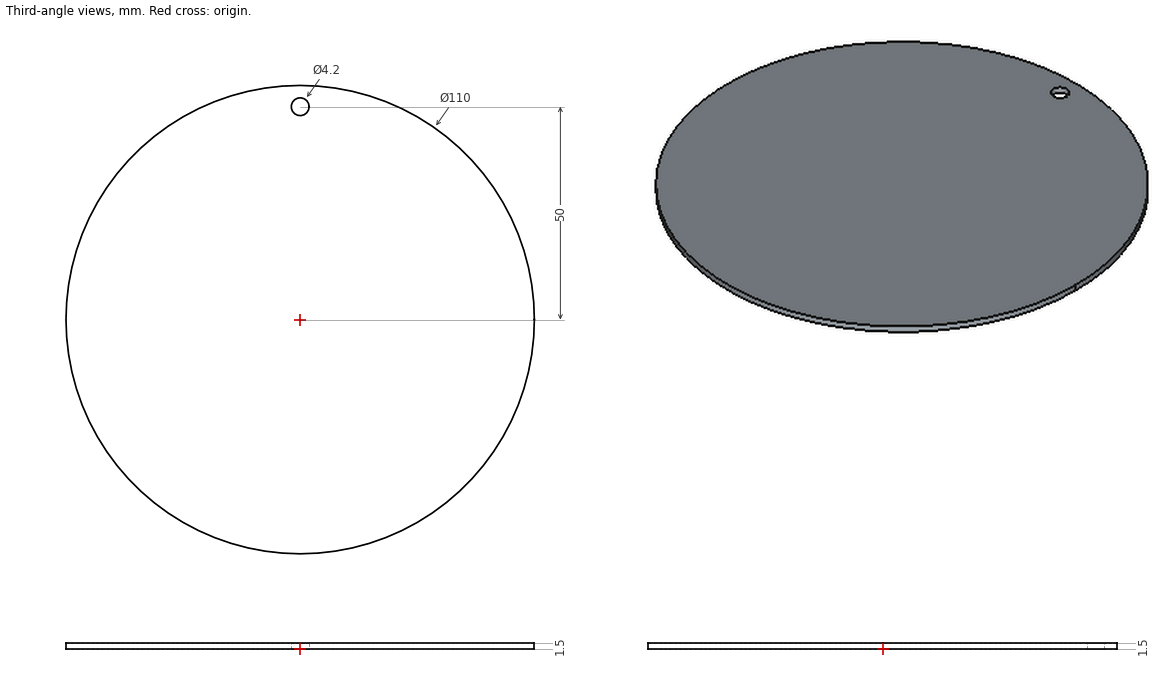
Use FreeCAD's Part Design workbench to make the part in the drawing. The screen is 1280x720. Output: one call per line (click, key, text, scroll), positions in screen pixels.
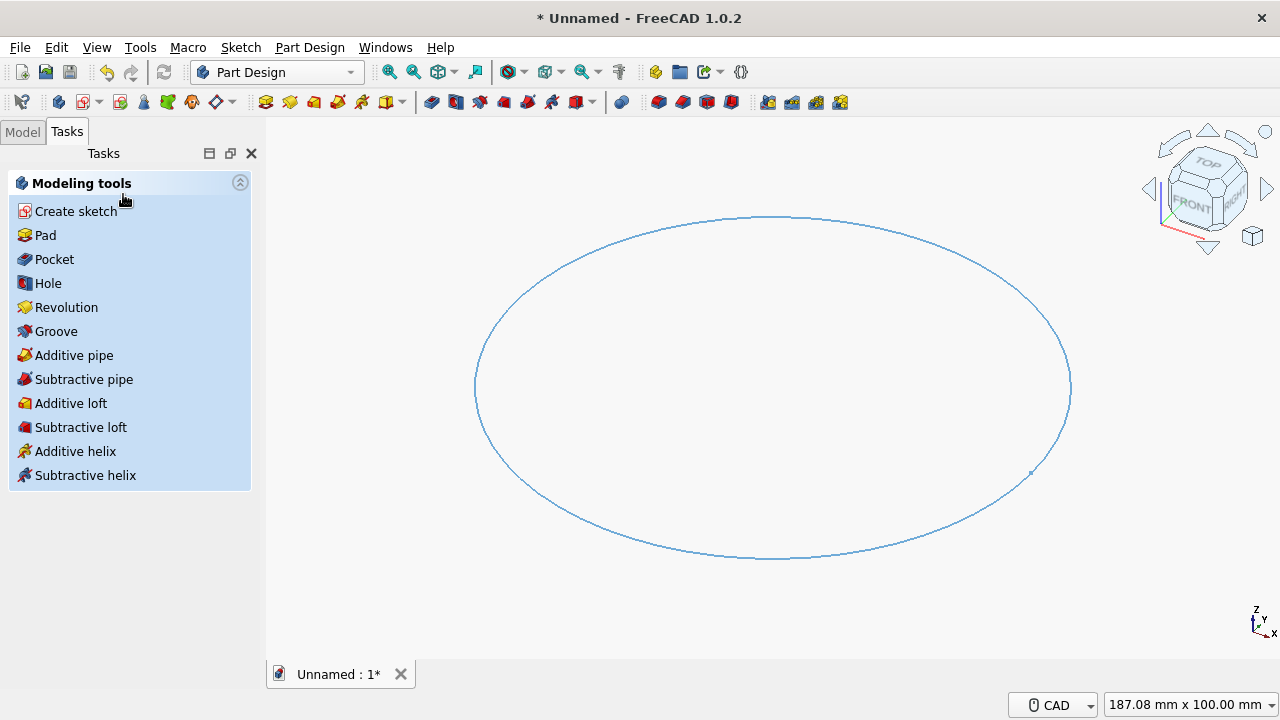
click(266, 102)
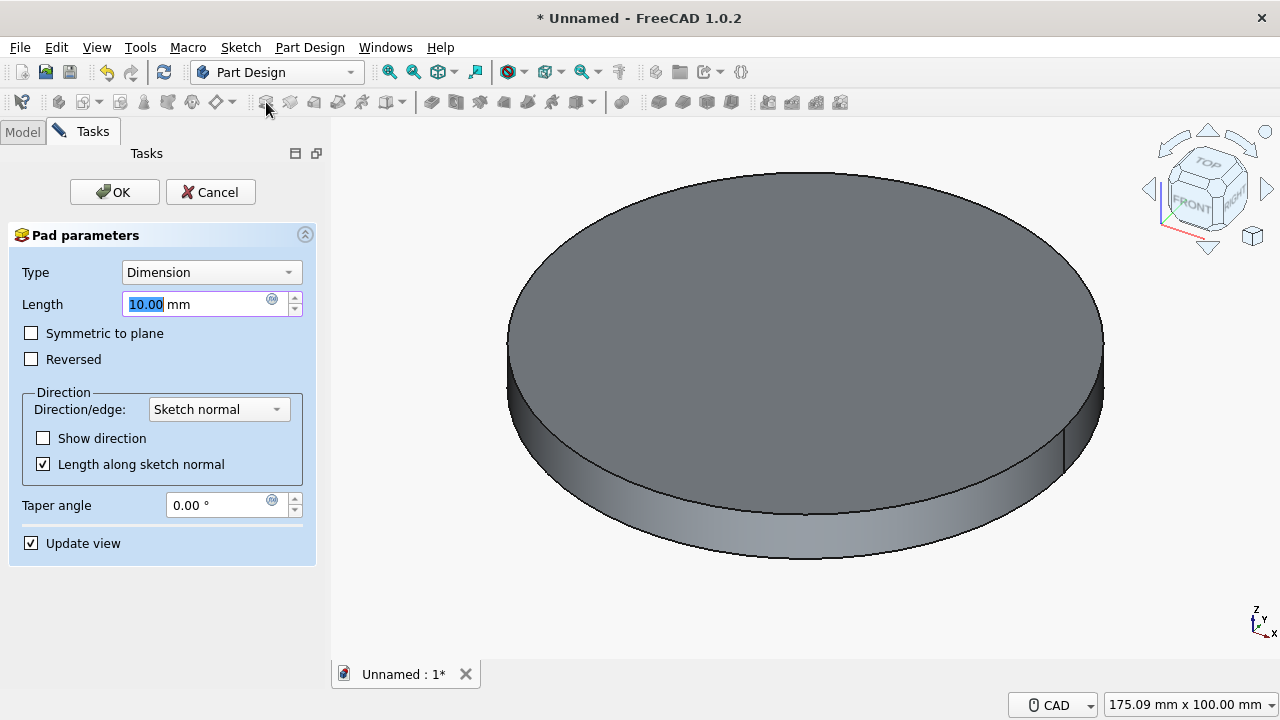
text(1.5)
key(Tab)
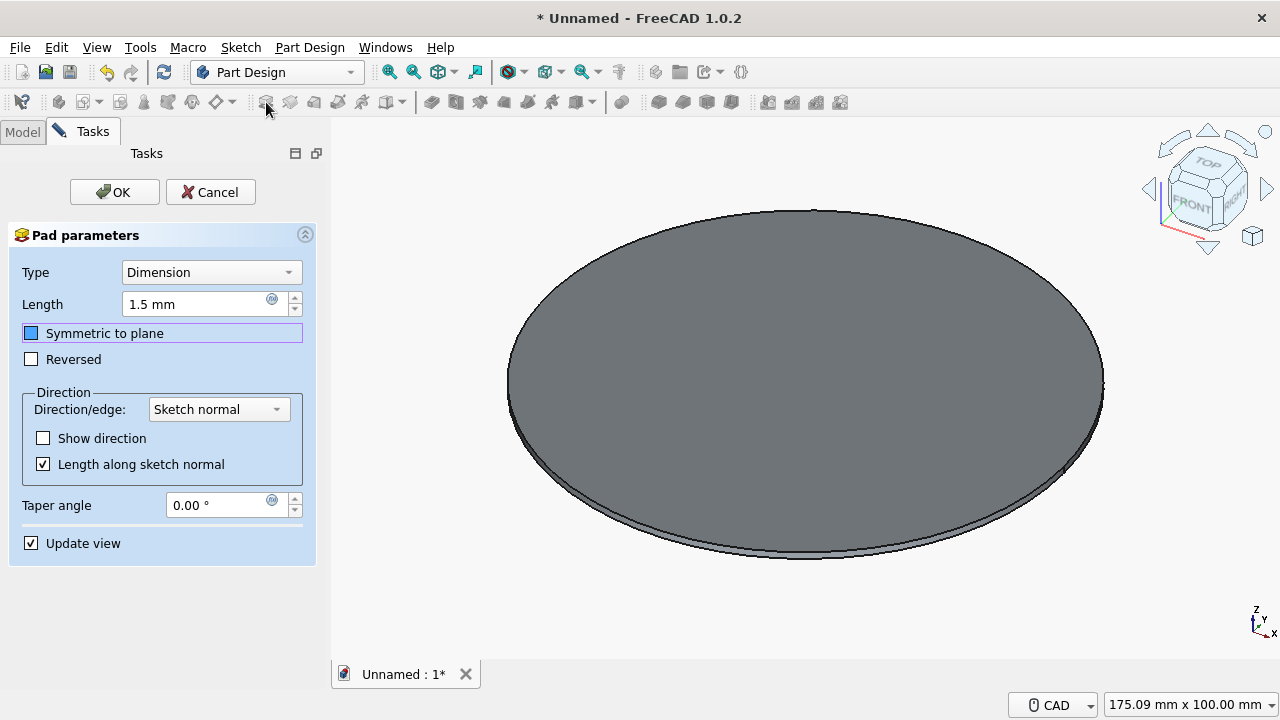
click(115, 192)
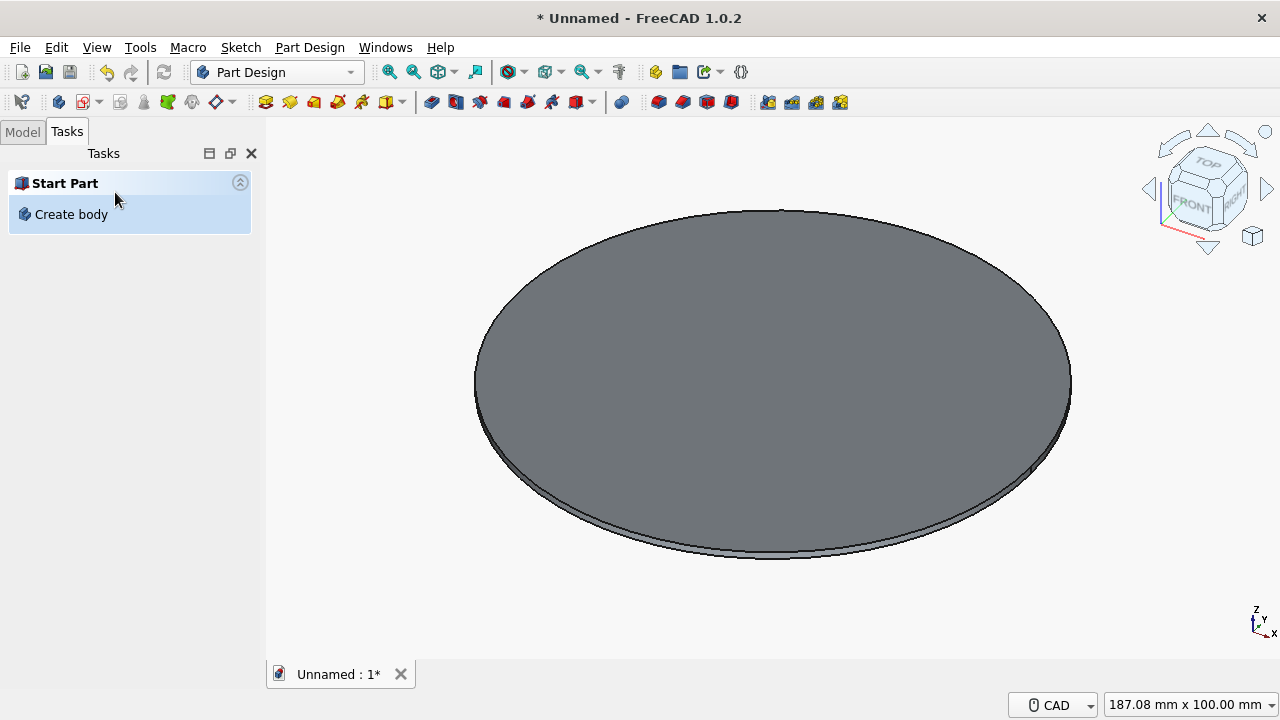
click(773, 380)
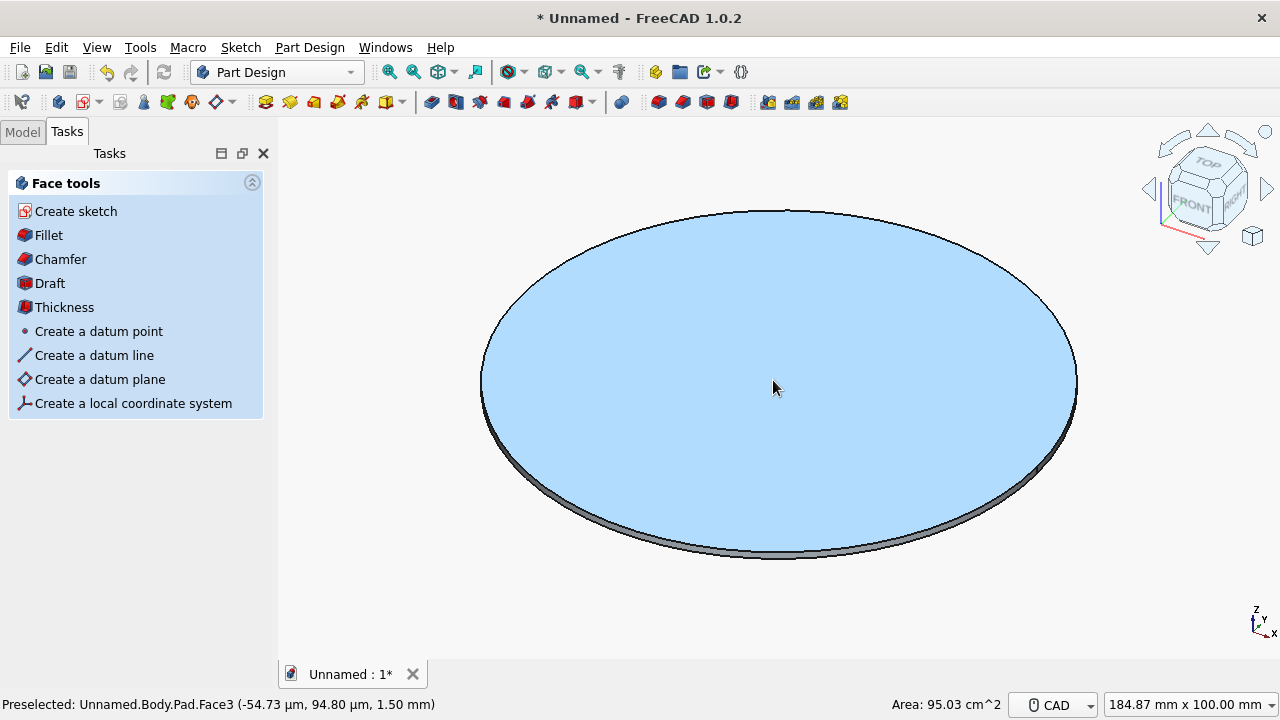
click(84, 102)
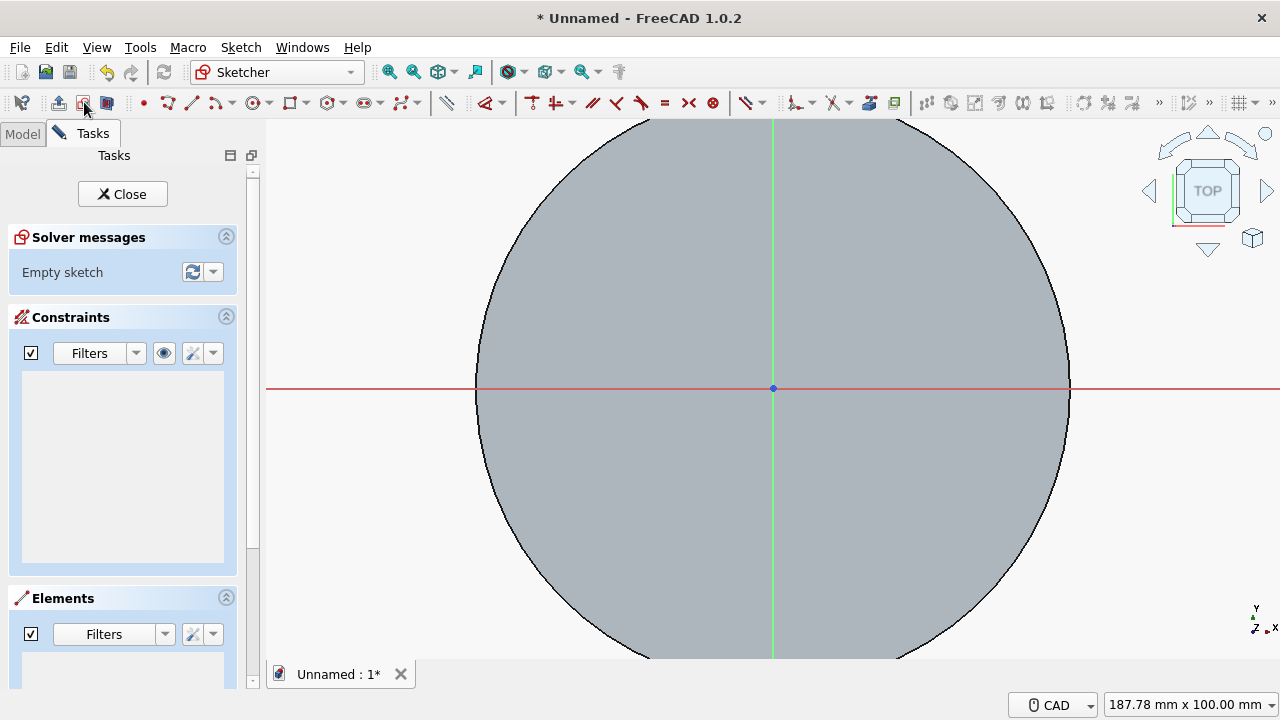
scroll(704, 389, down, 5)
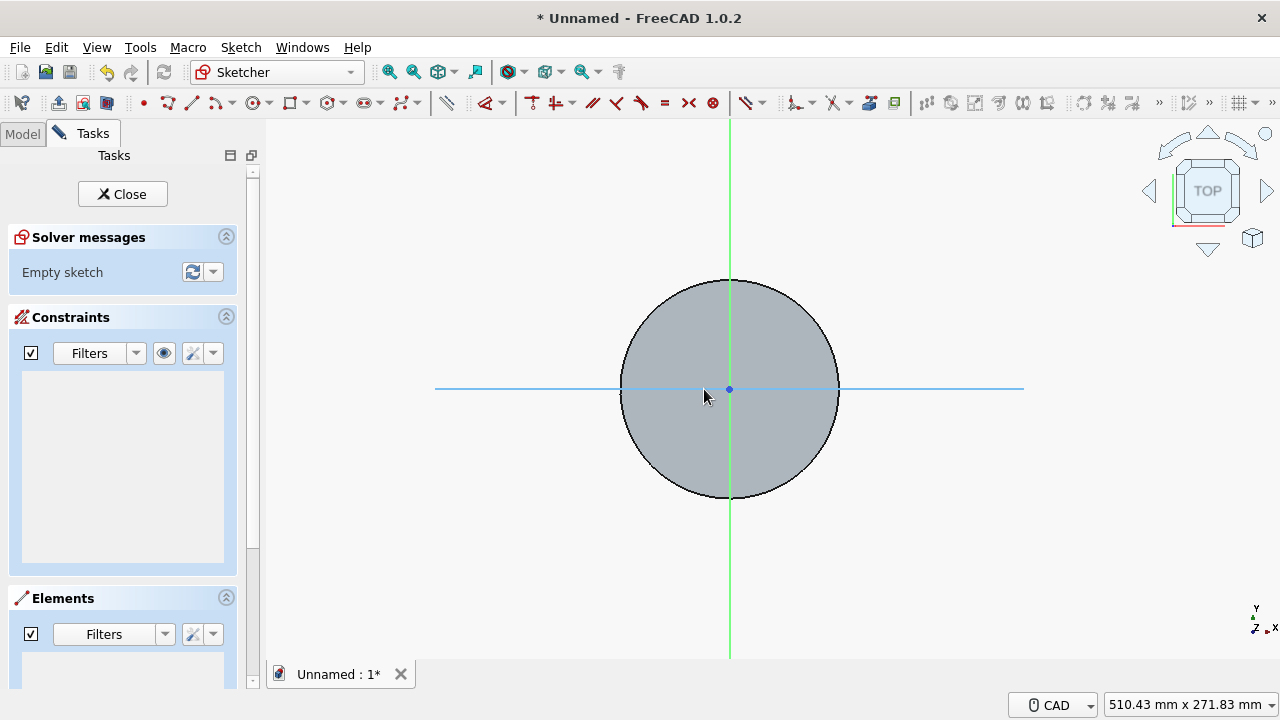
scroll(731, 285, up, 15)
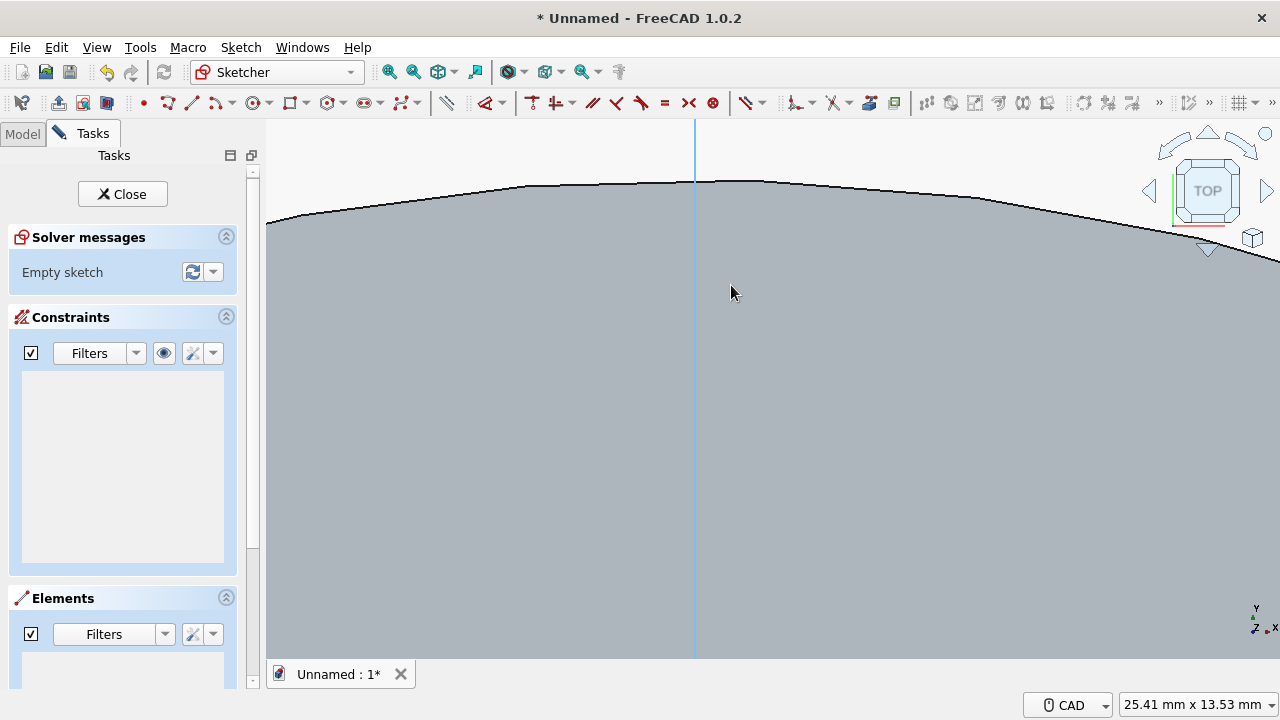
scroll(688, 371, up, 4)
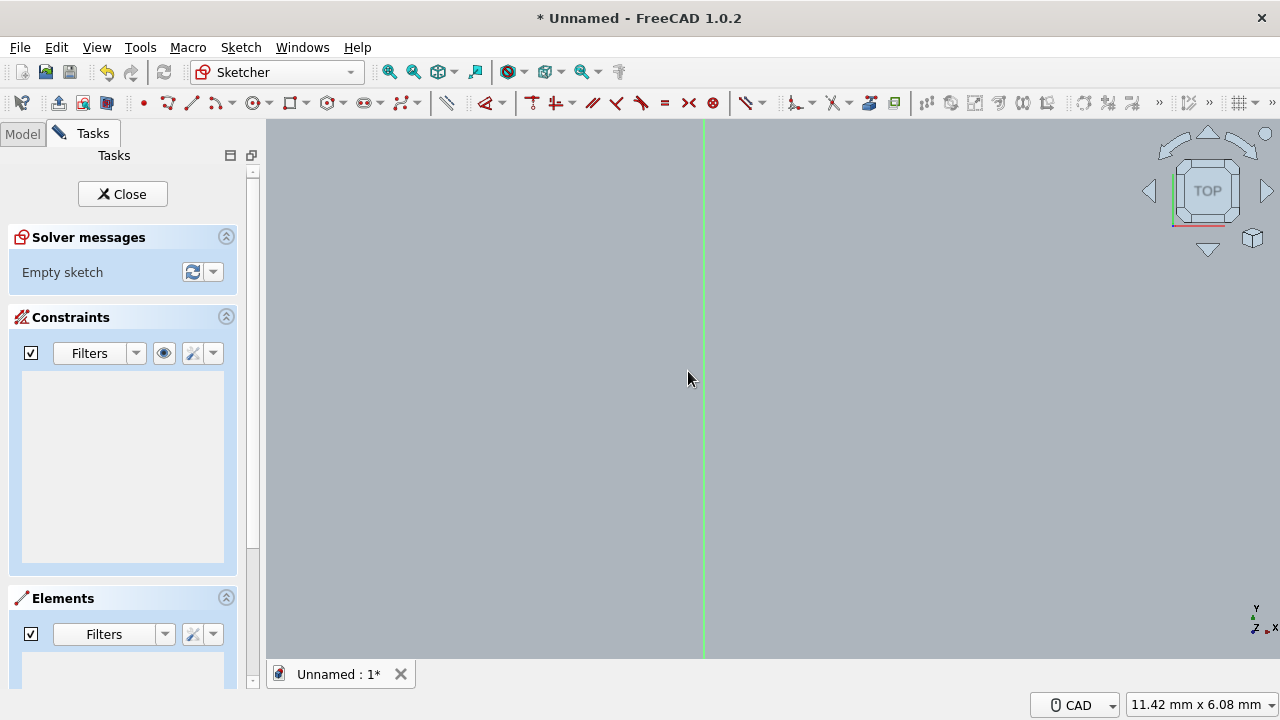
click(254, 104)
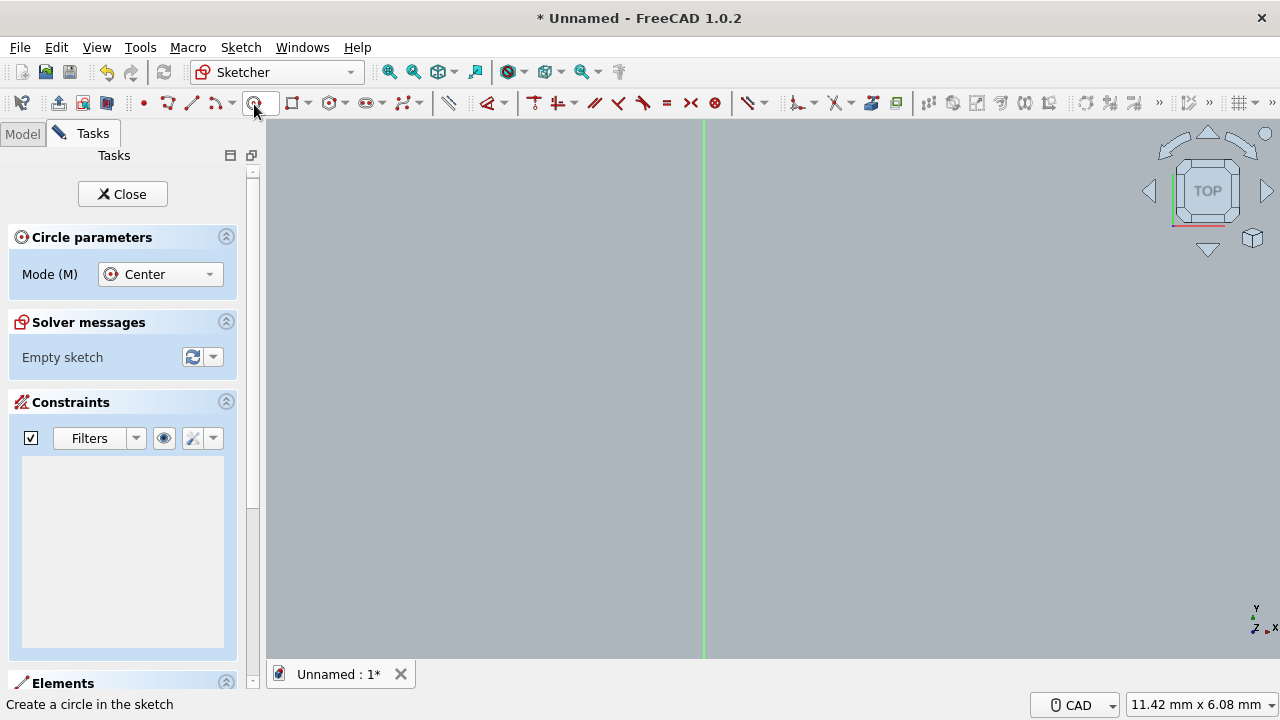
click(704, 389)
click(836, 257)
key(Escape)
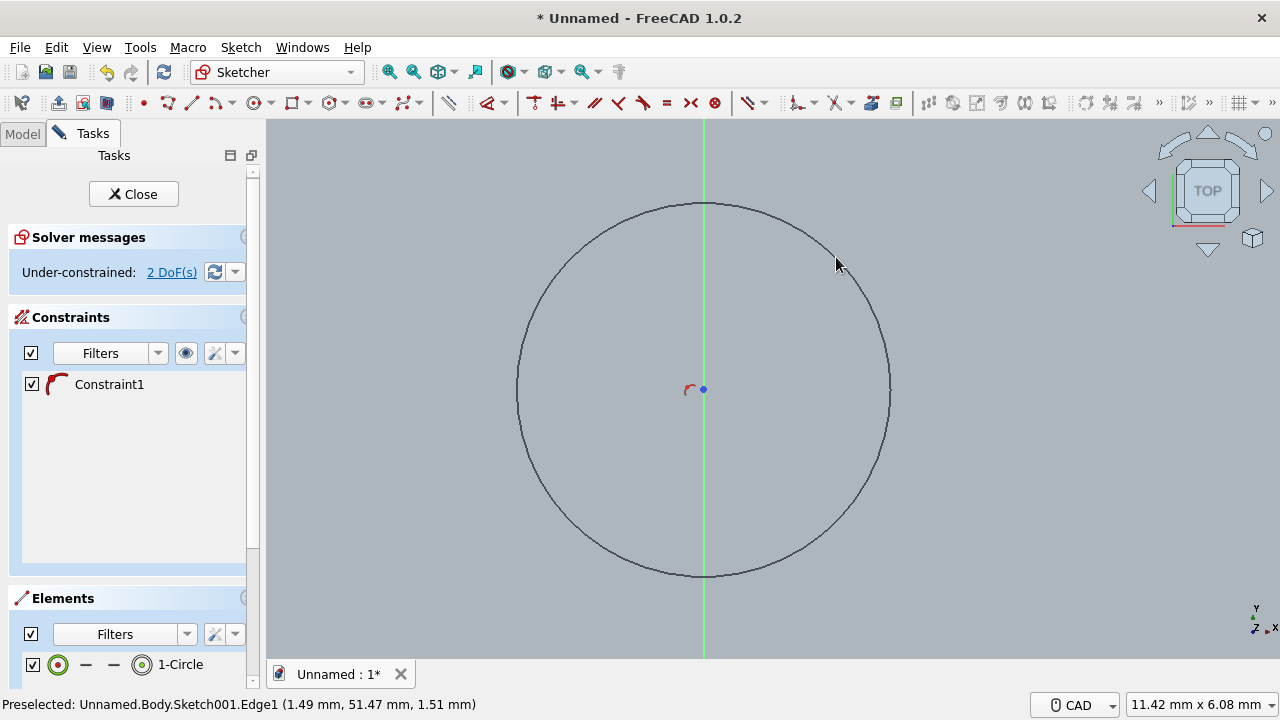
click(488, 104)